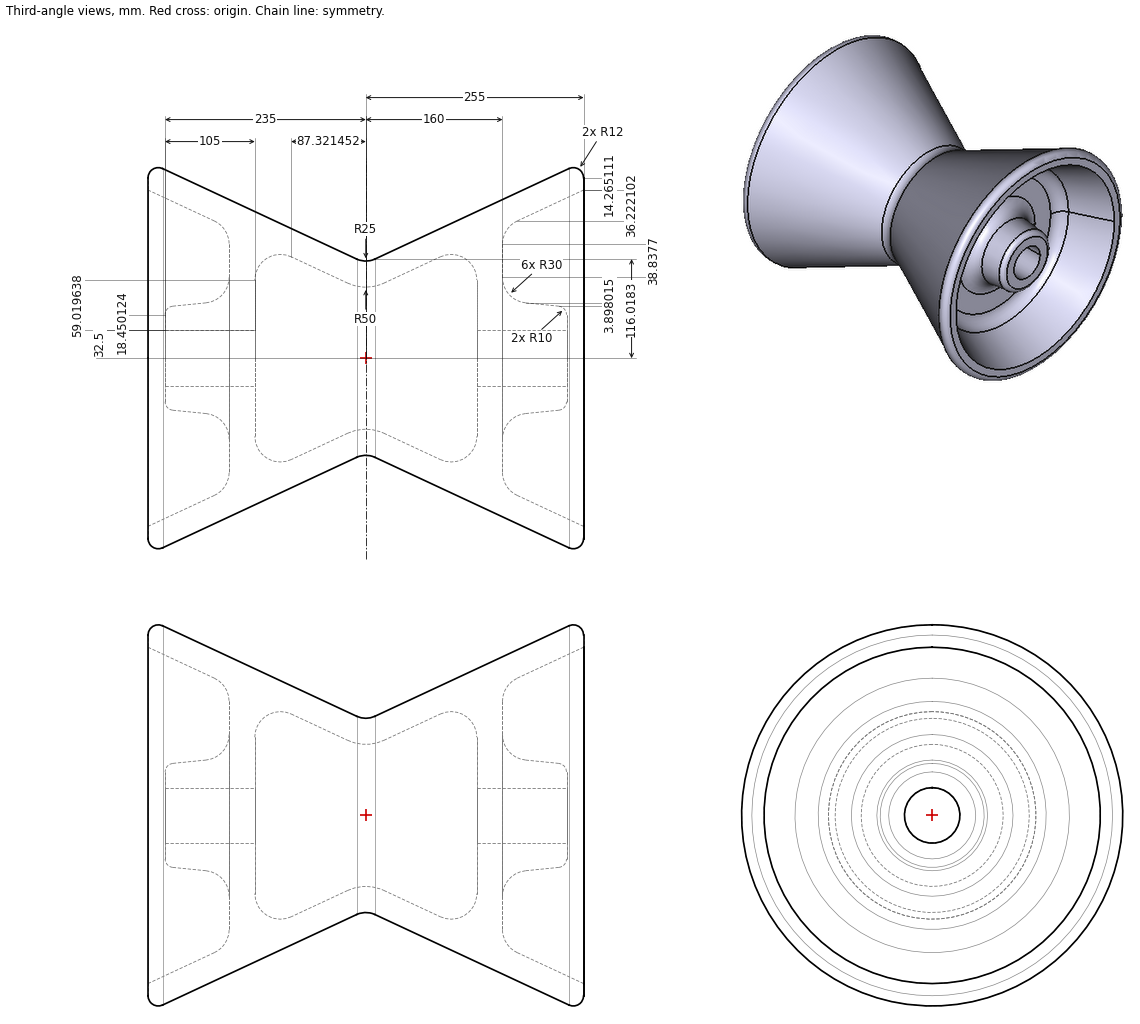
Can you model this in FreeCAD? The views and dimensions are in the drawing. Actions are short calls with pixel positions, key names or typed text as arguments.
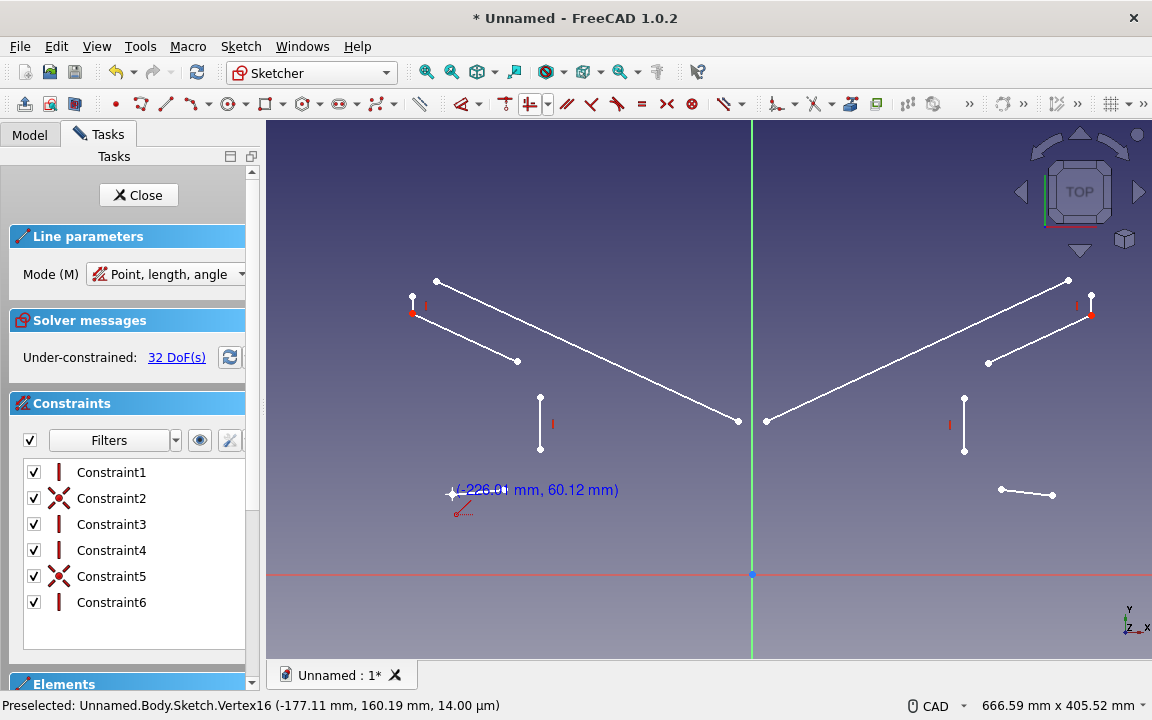
click(141, 104)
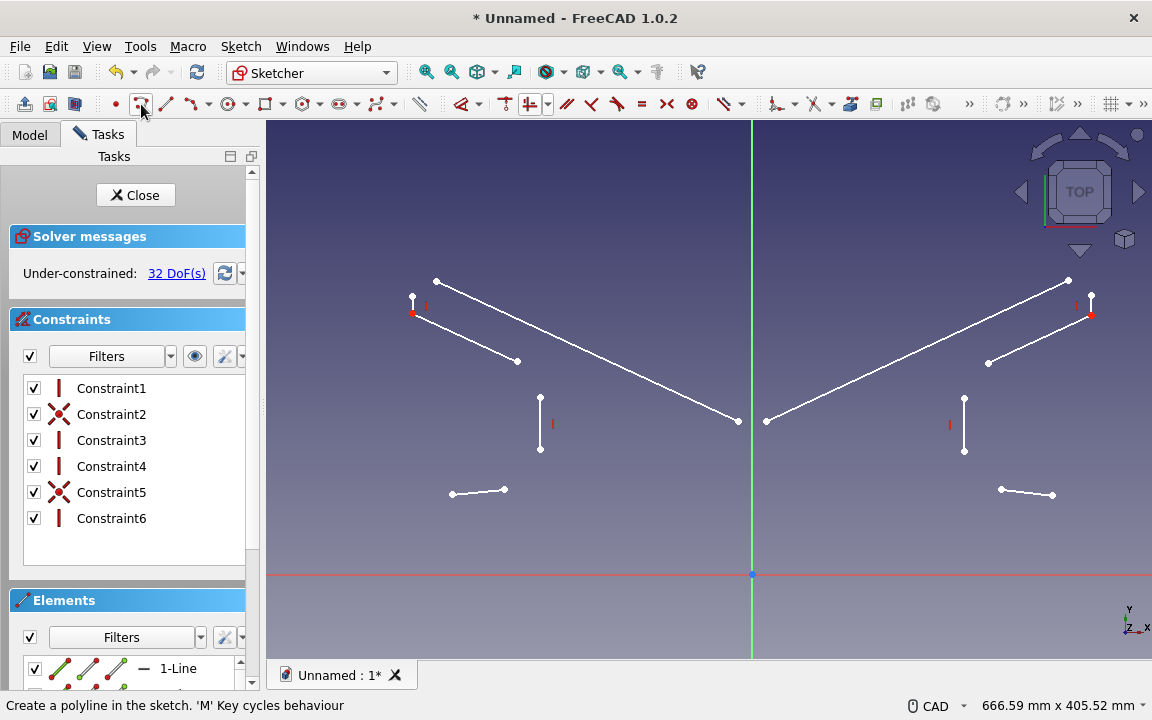
click(440, 507)
click(440, 532)
click(580, 532)
click(580, 453)
right_click(580, 453)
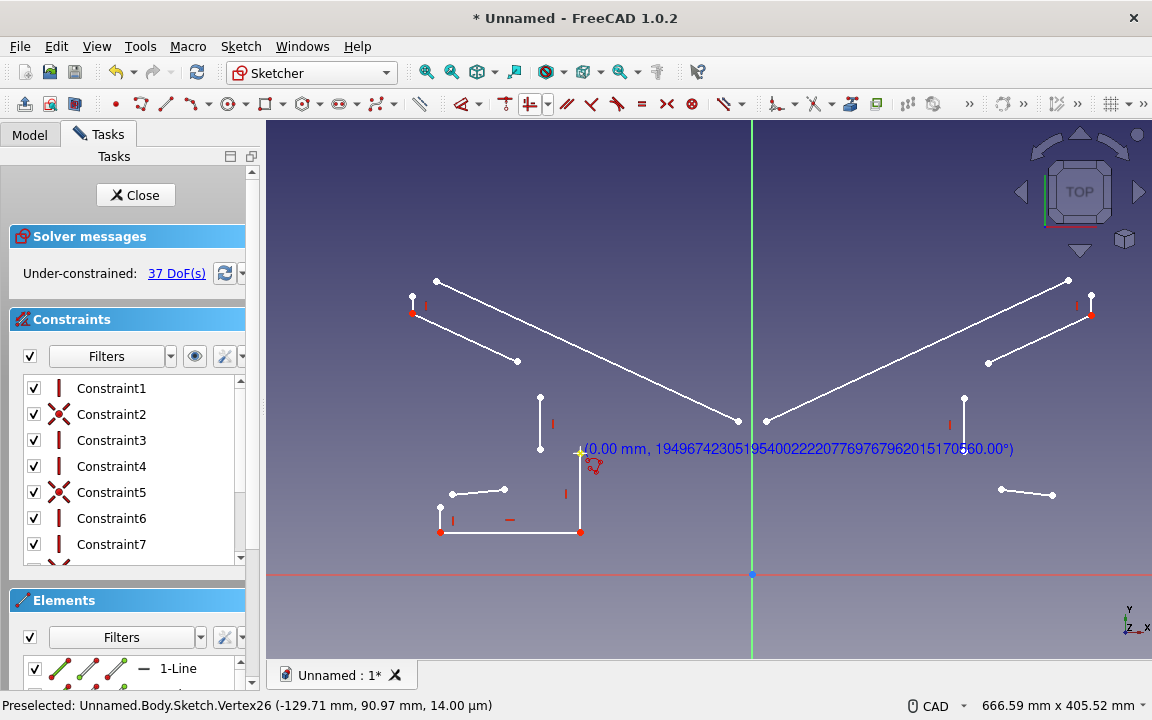
click(166, 104)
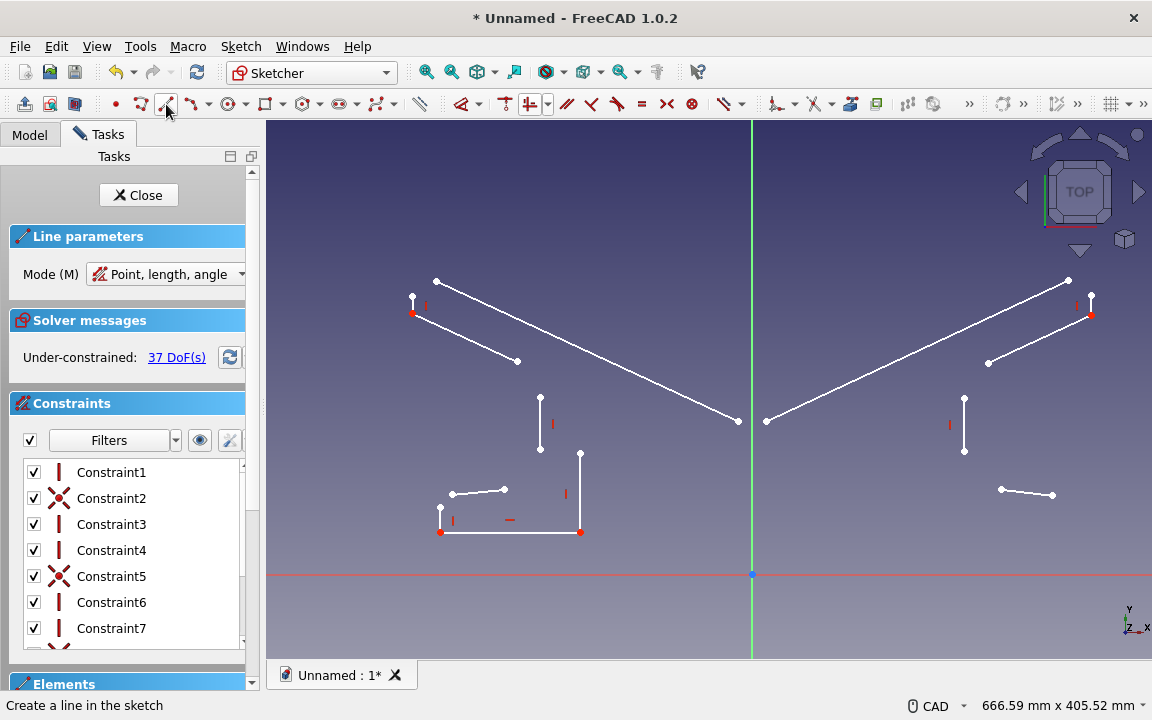
click(636, 417)
click(724, 458)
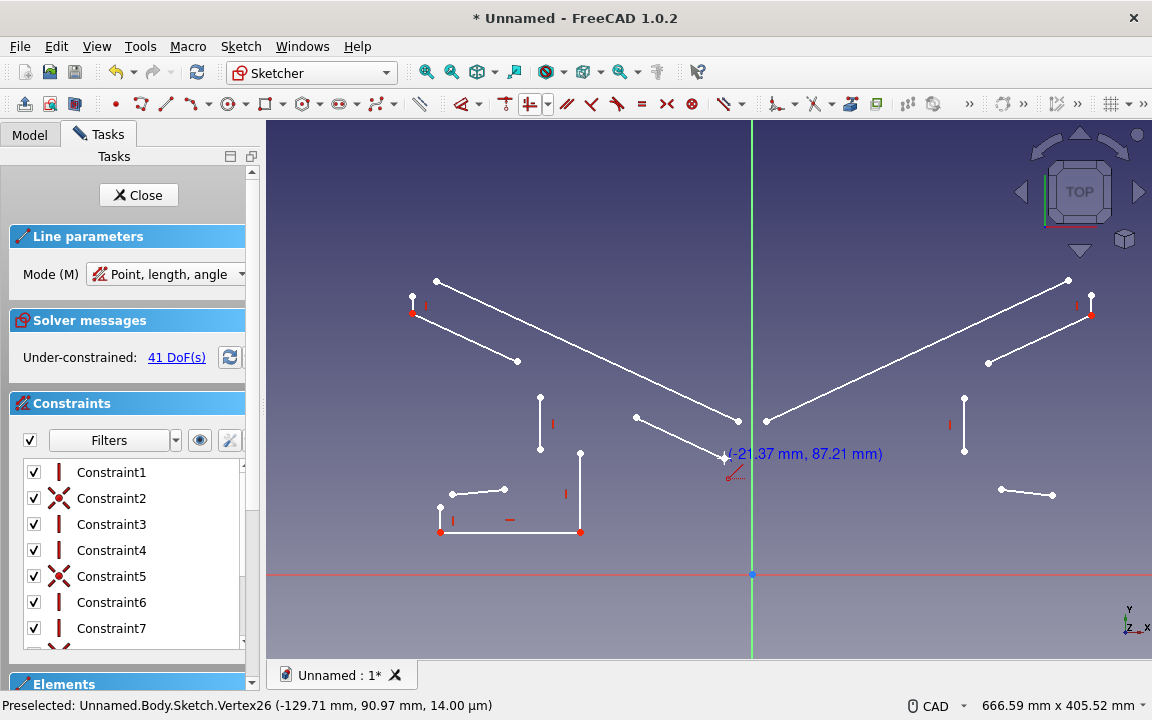
click(780, 458)
click(868, 417)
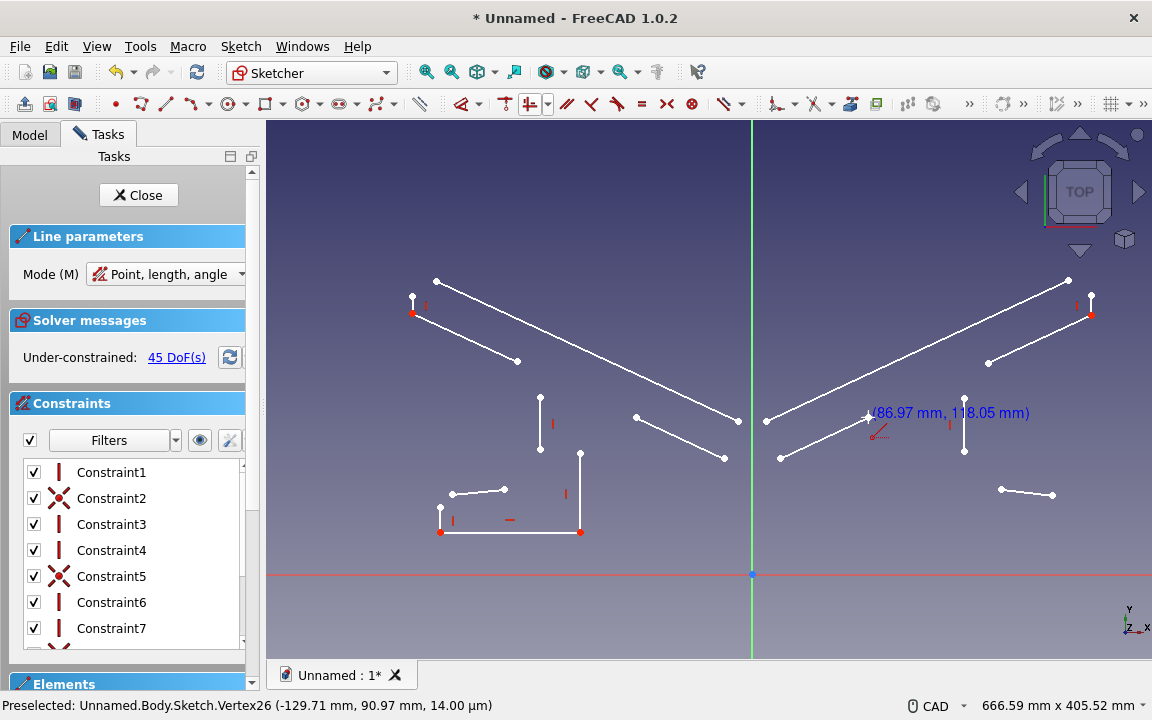
click(141, 104)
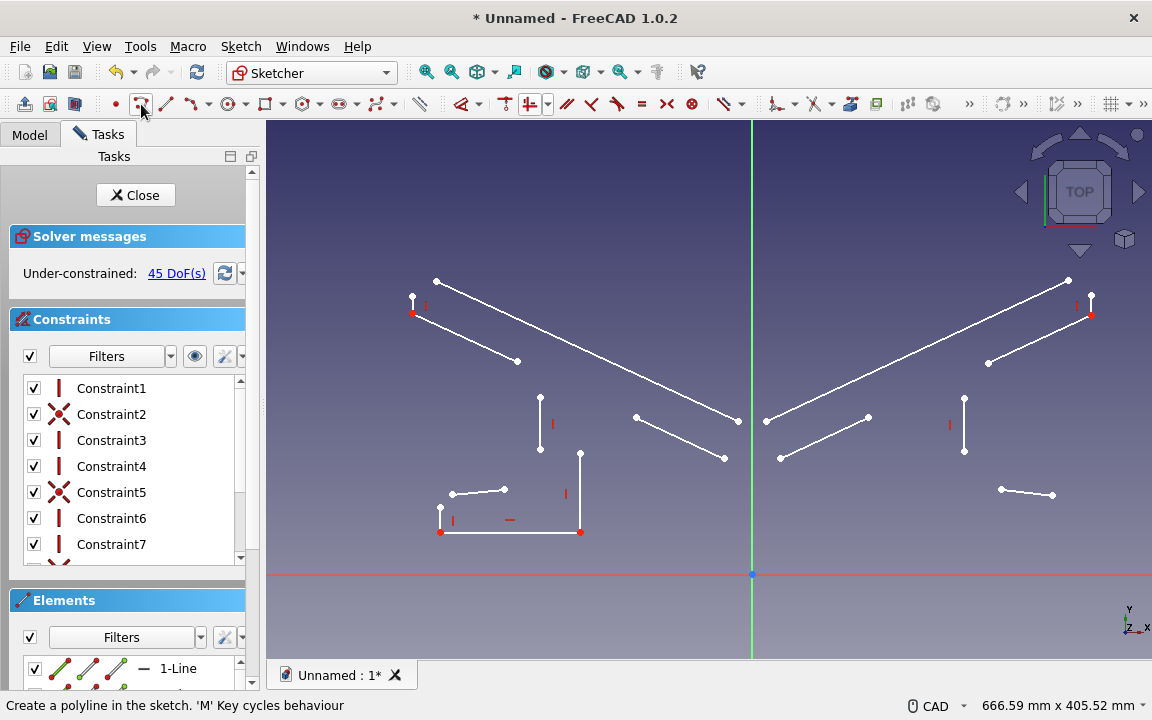
click(925, 453)
click(925, 532)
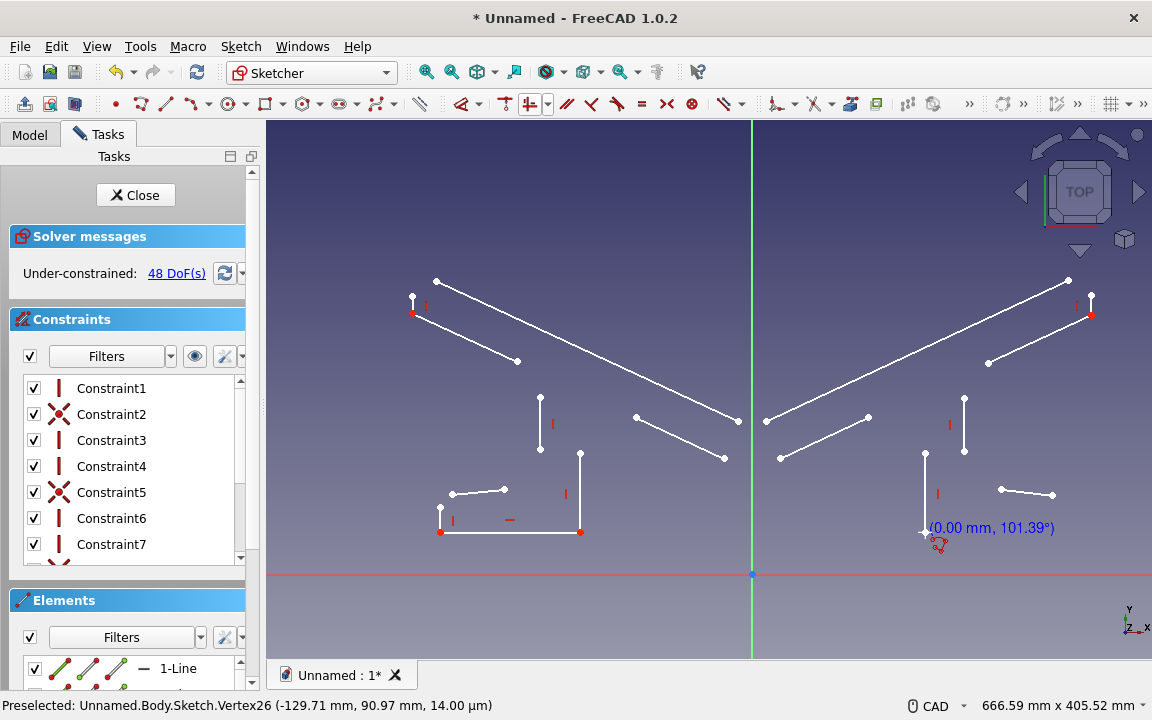
scroll(413, 313, down, 2)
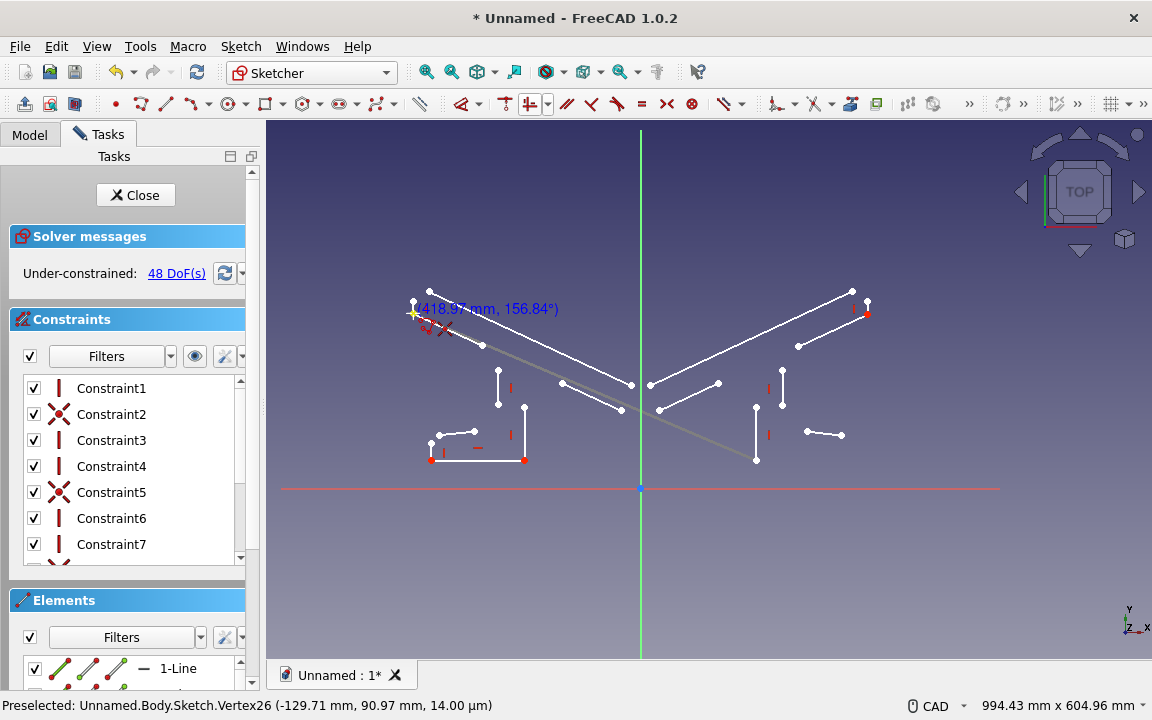
click(850, 460)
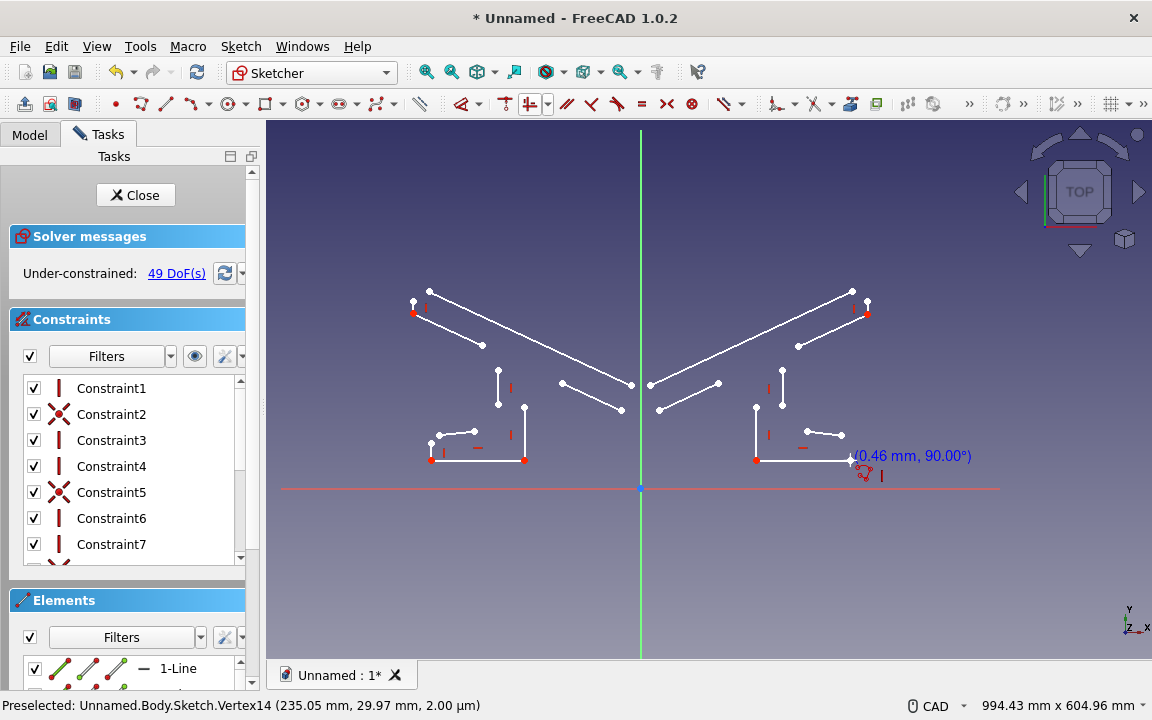
scroll(850, 443, up, 2)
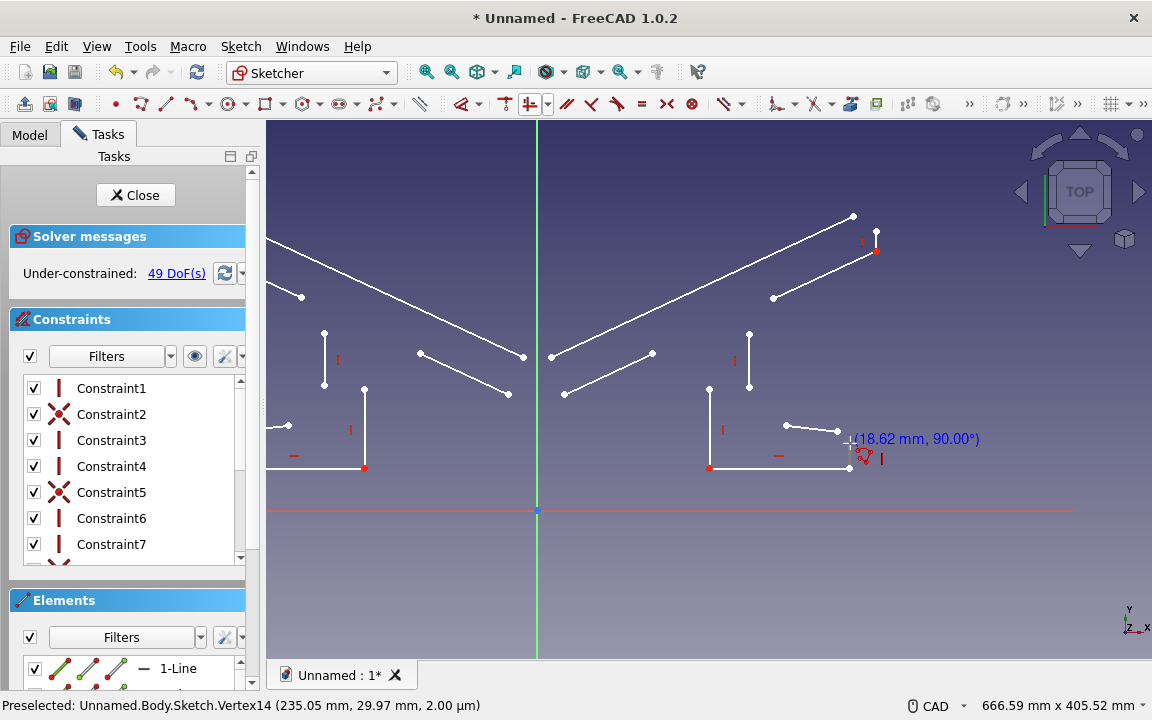
click(850, 443)
right_click(850, 443)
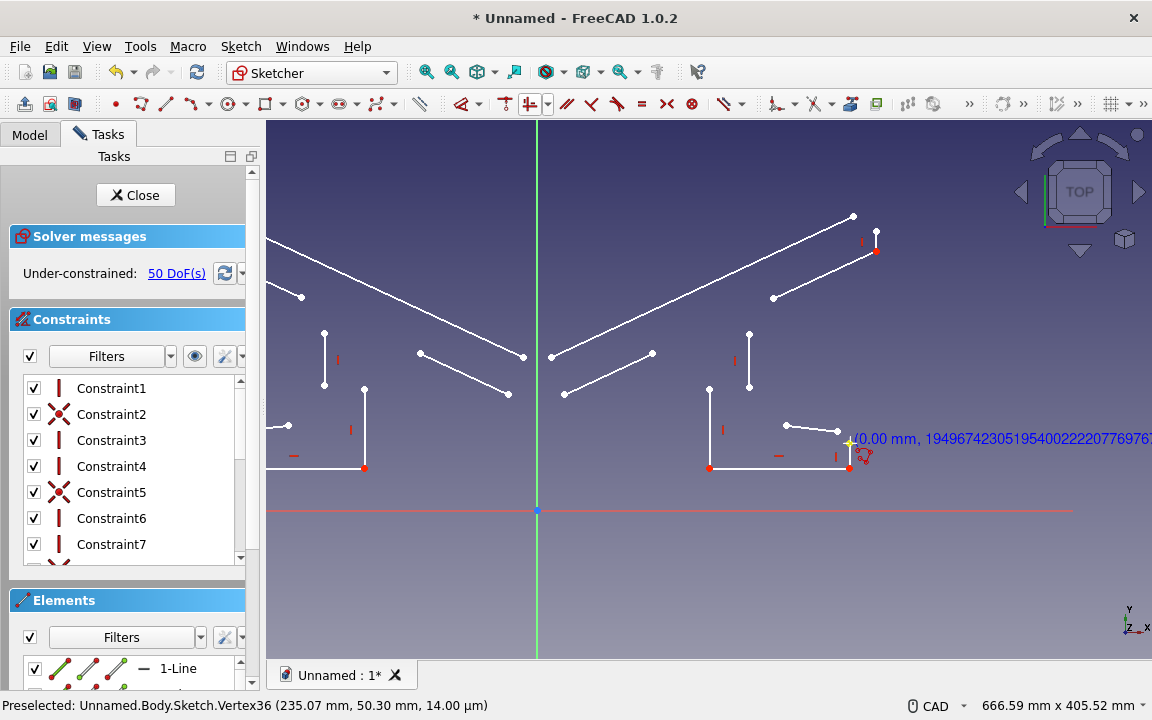
click(190, 104)